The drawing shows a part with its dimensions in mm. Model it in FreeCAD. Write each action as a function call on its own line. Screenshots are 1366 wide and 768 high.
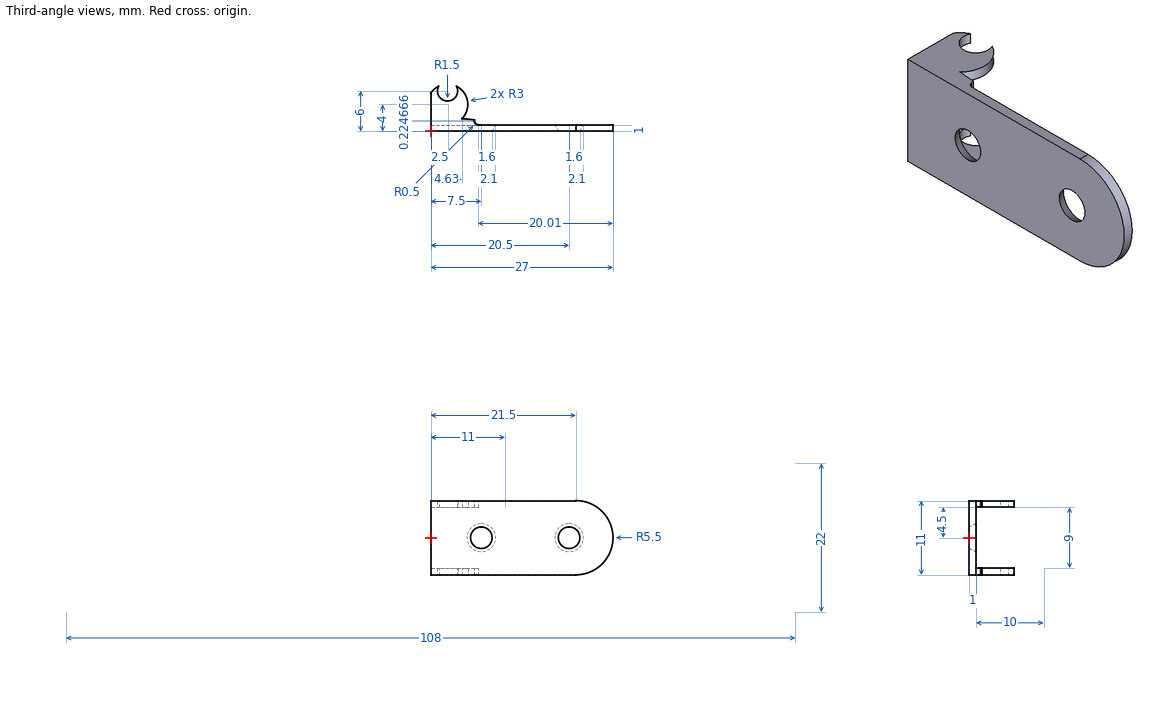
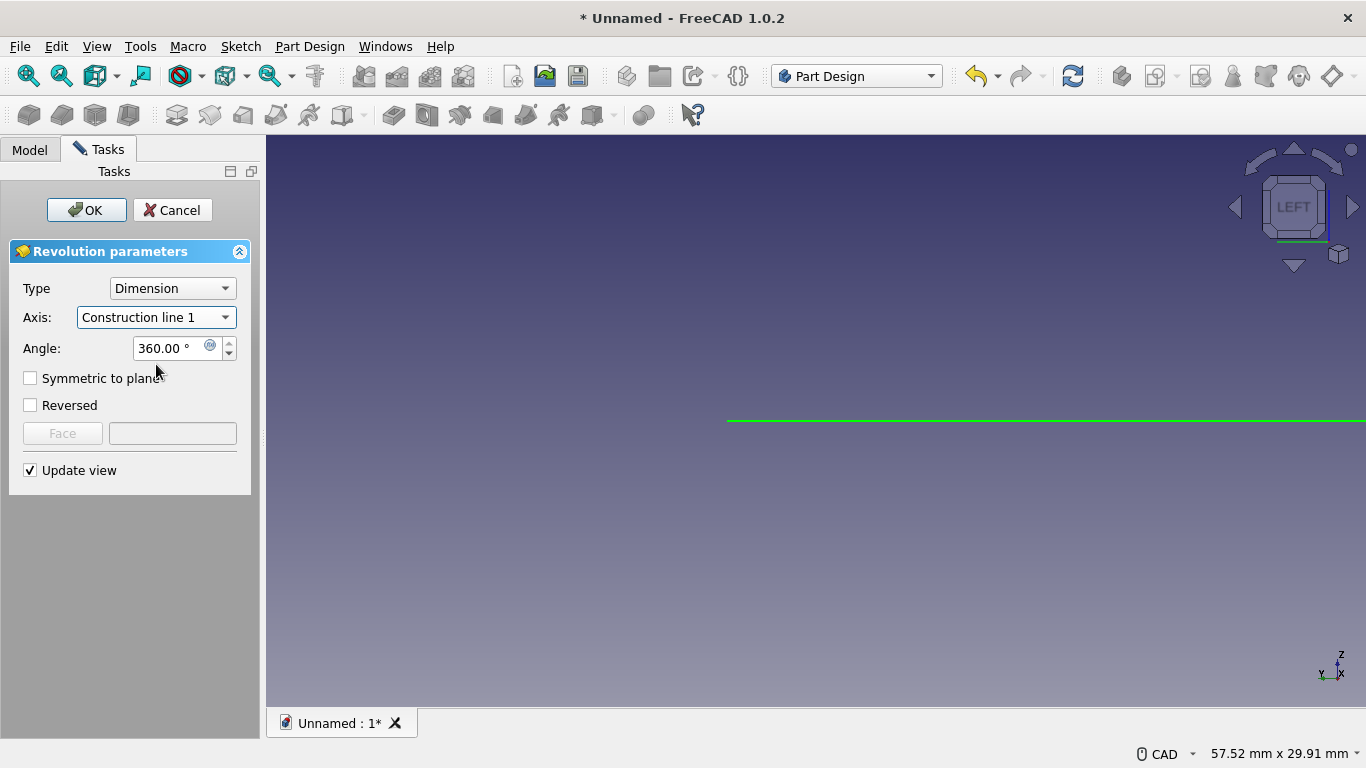
click(87, 210)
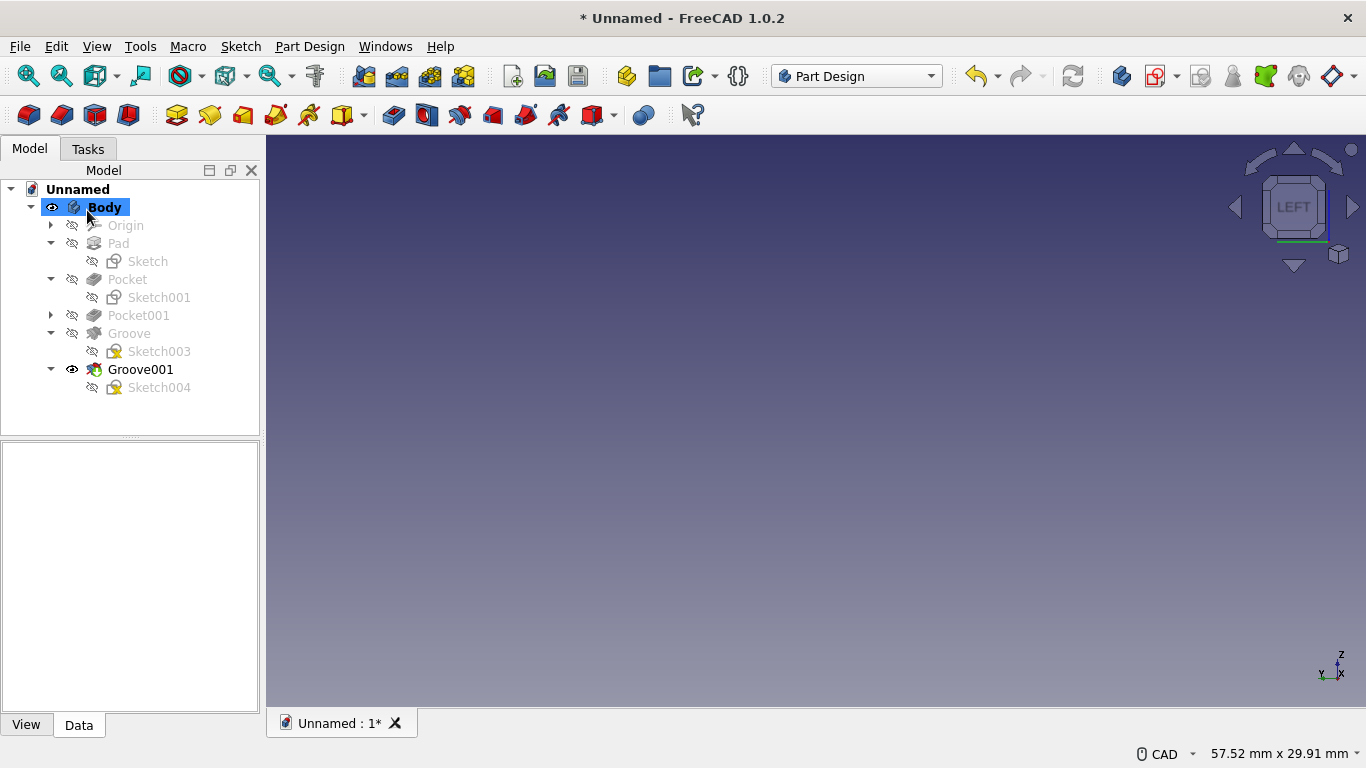
key(0)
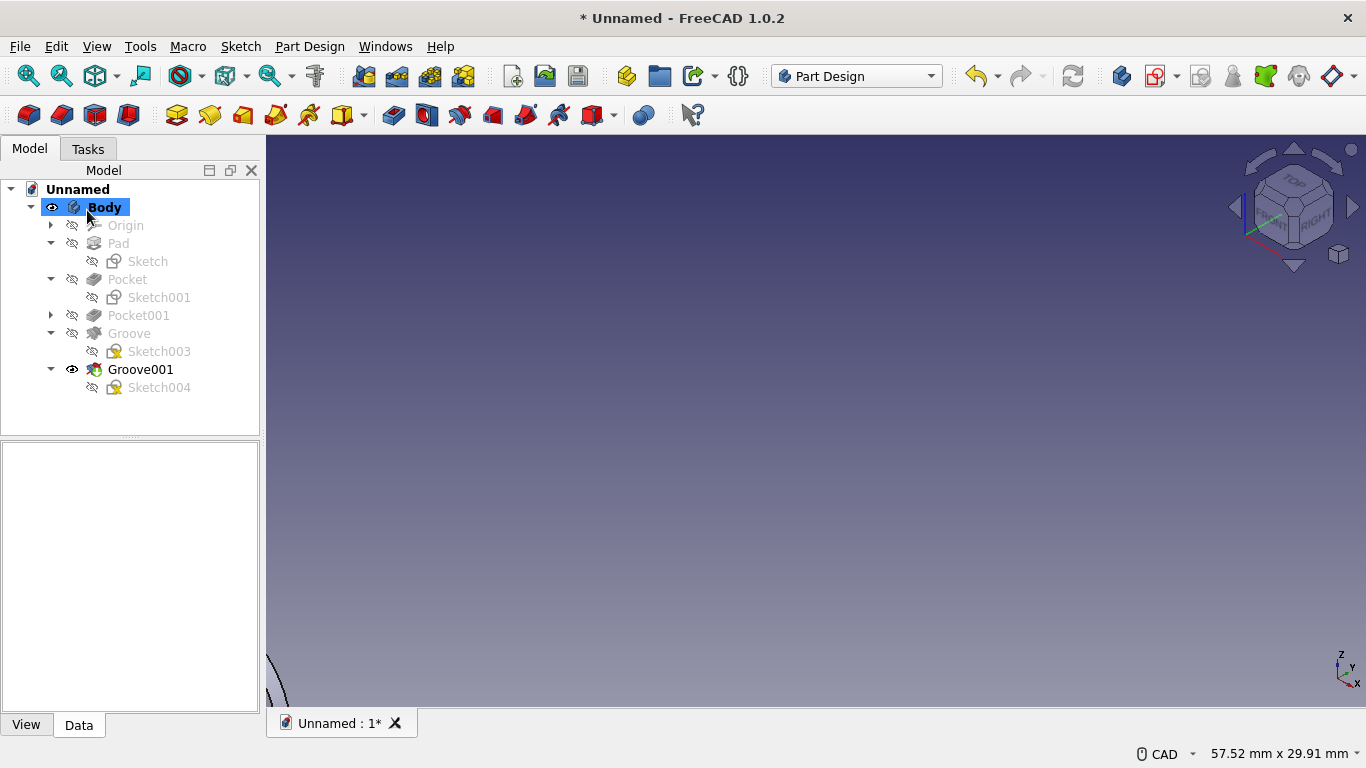
key(v)
key(f)